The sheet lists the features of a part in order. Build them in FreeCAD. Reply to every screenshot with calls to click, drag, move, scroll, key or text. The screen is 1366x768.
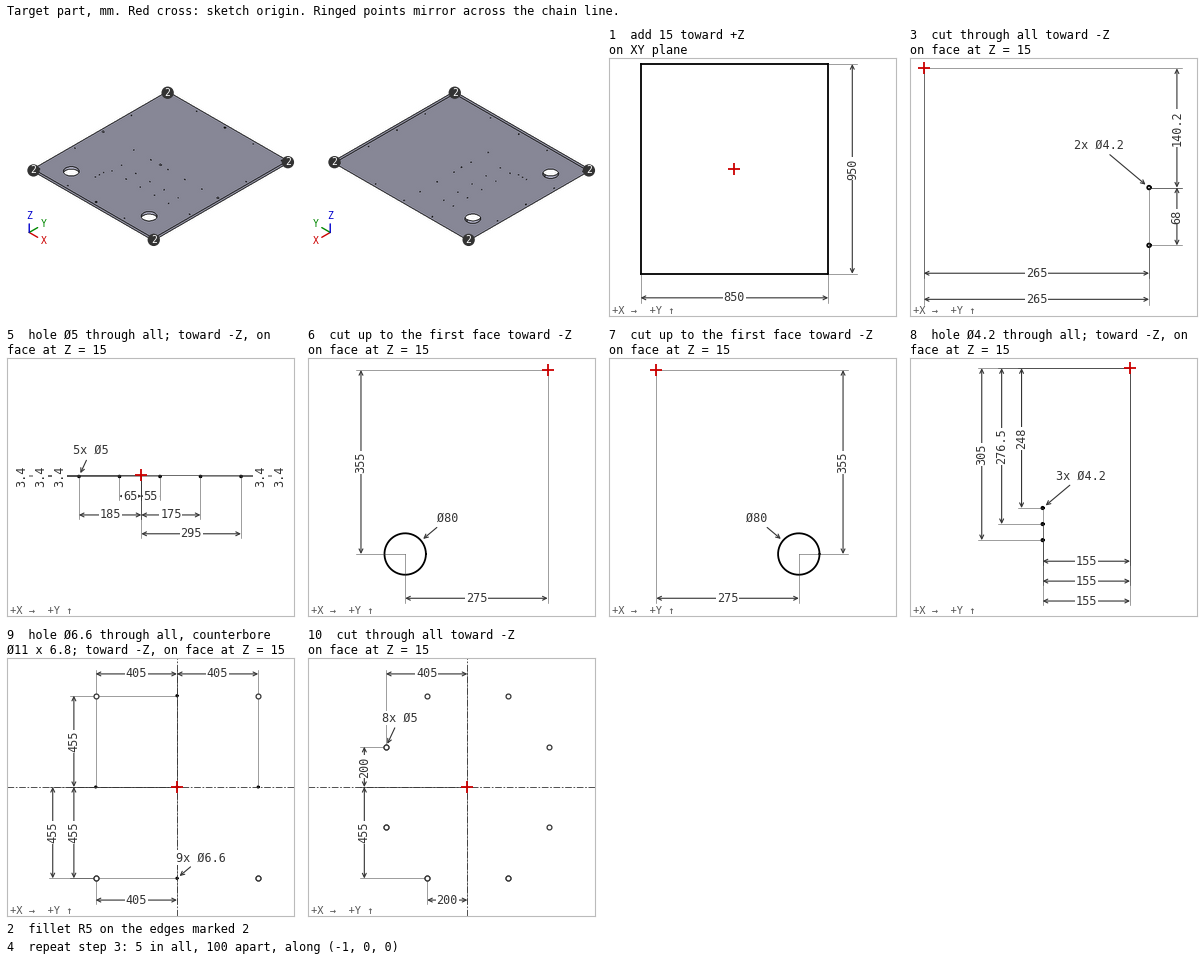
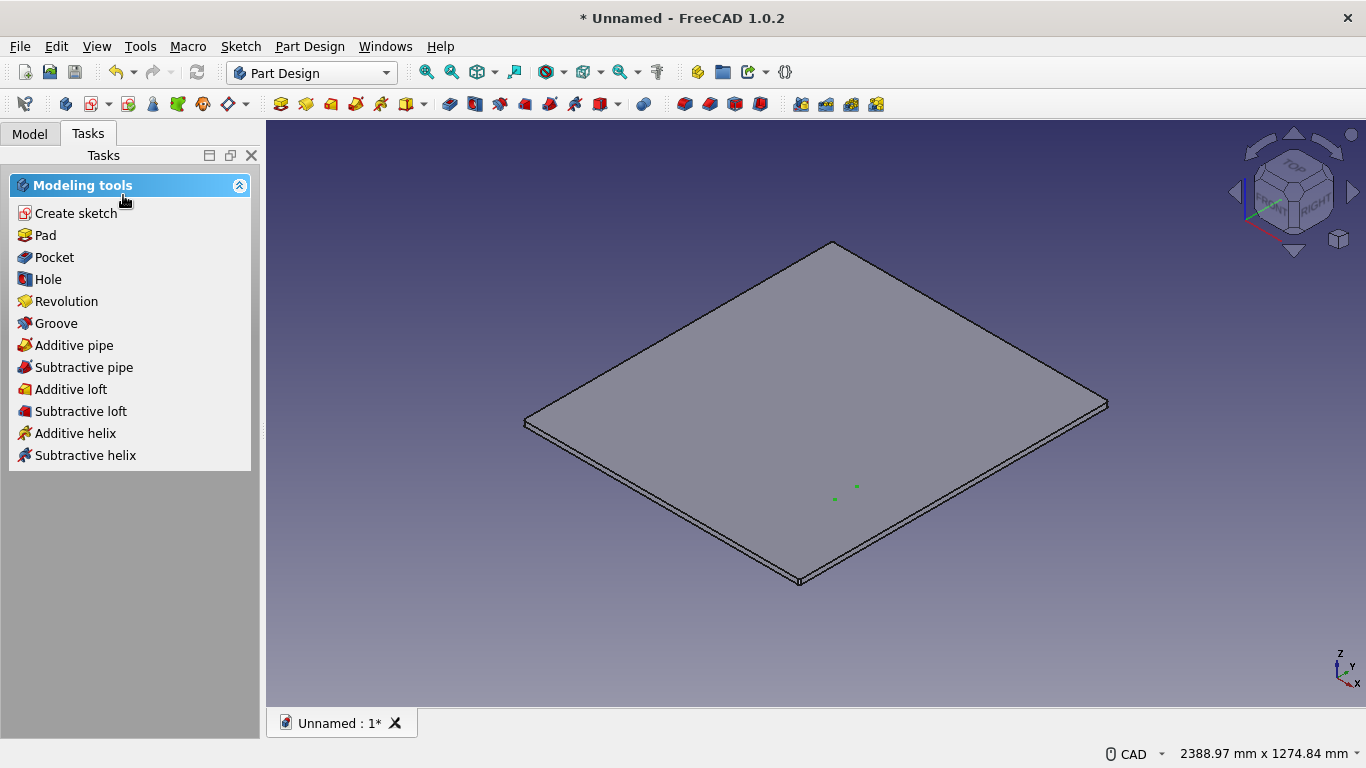
click(450, 104)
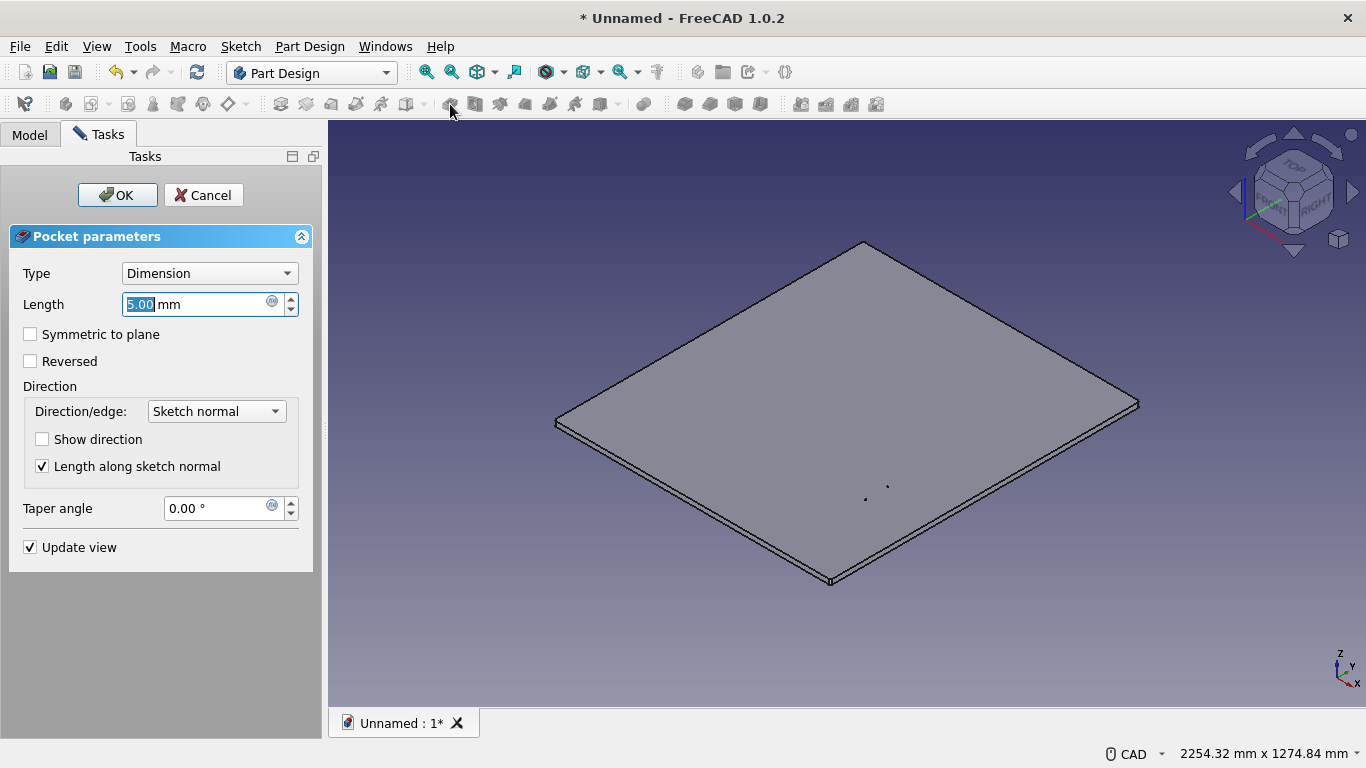
click(210, 274)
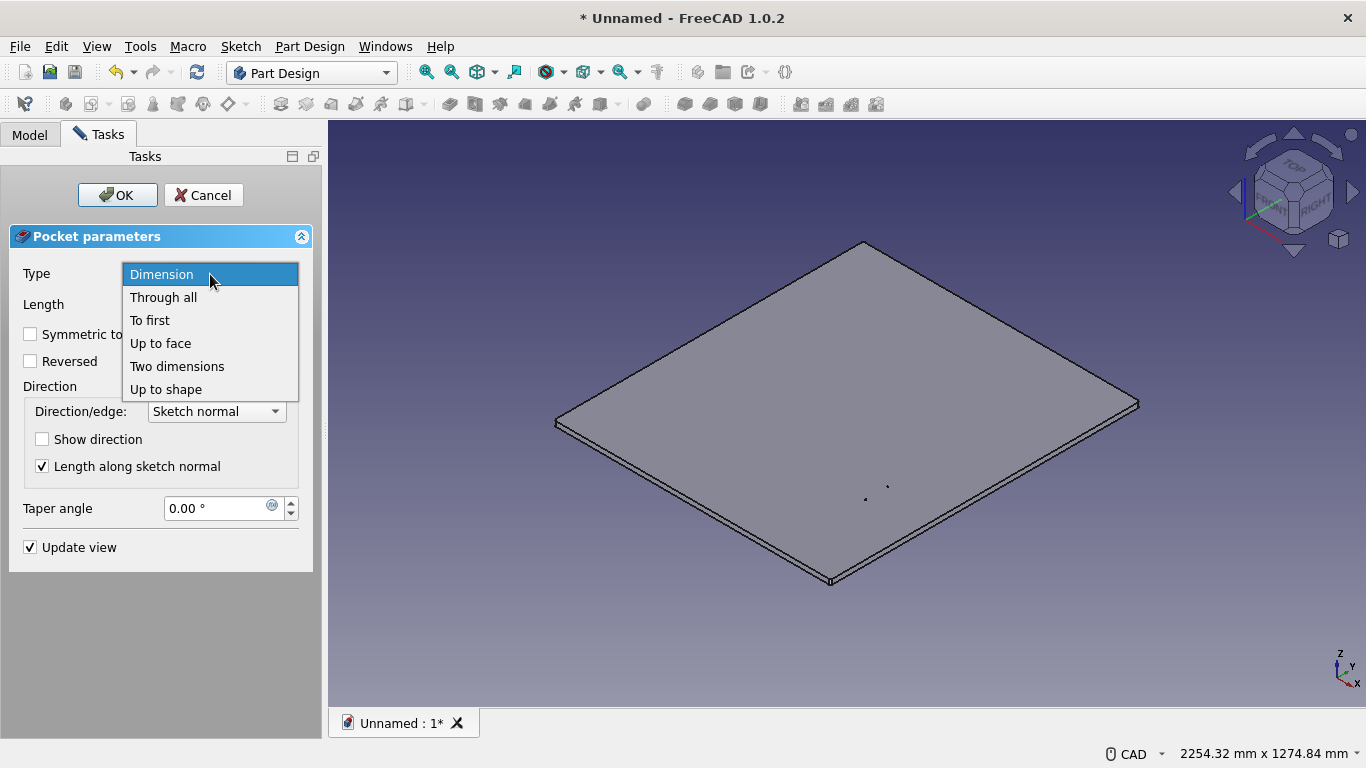
click(208, 298)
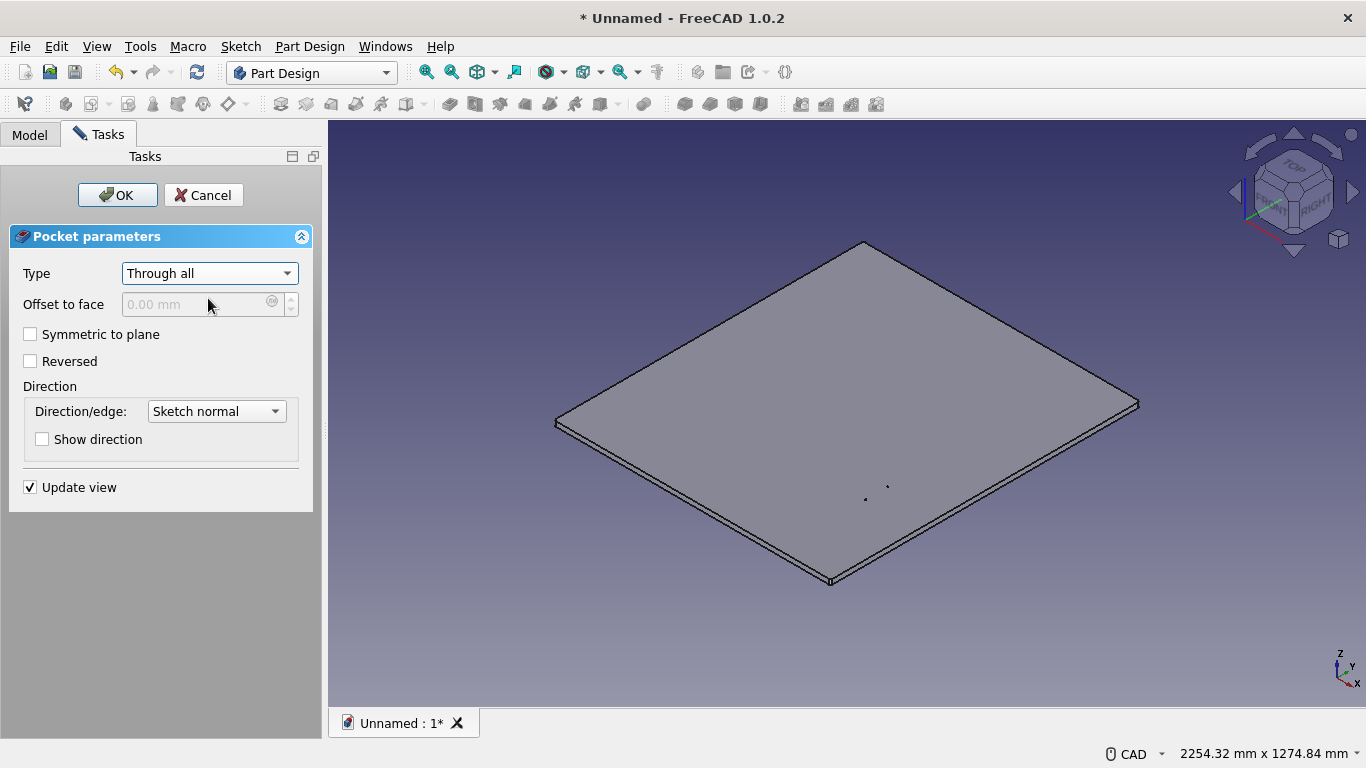
click(118, 195)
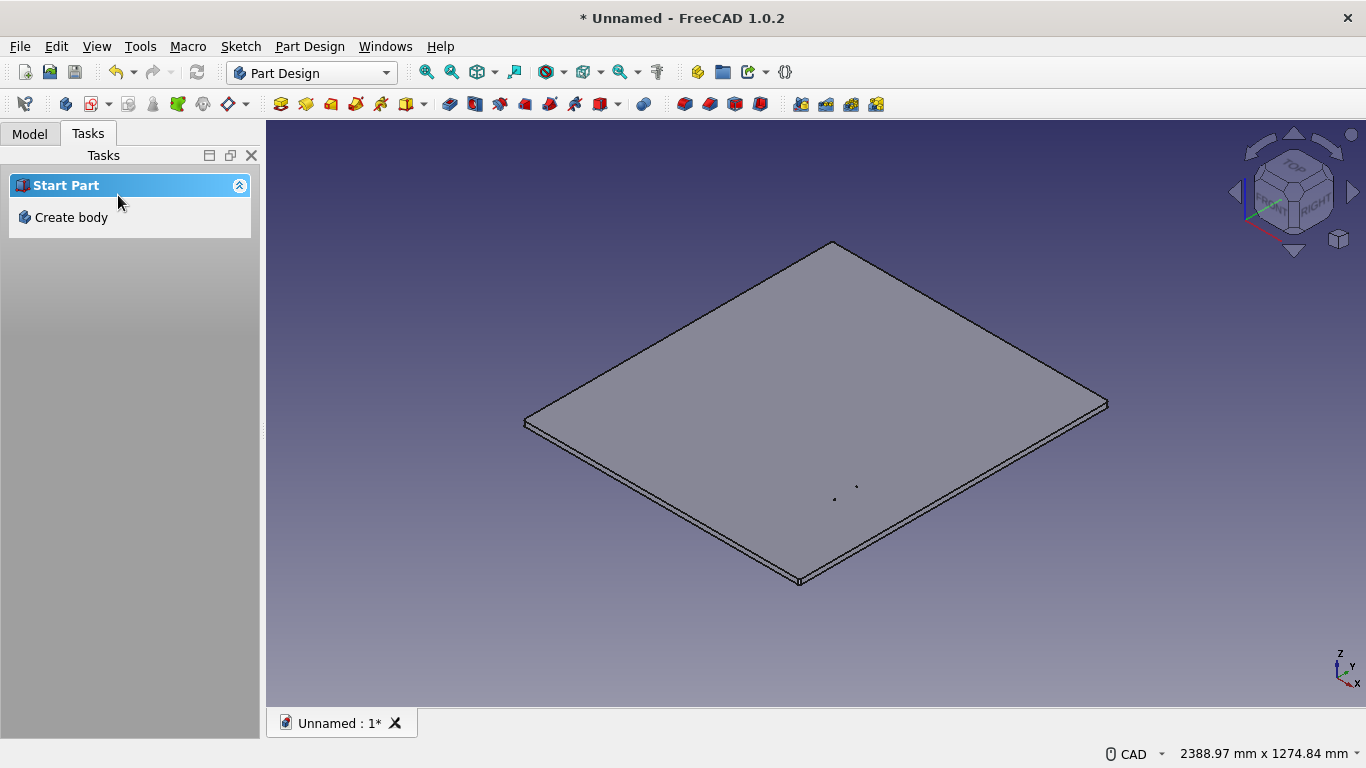
click(30, 134)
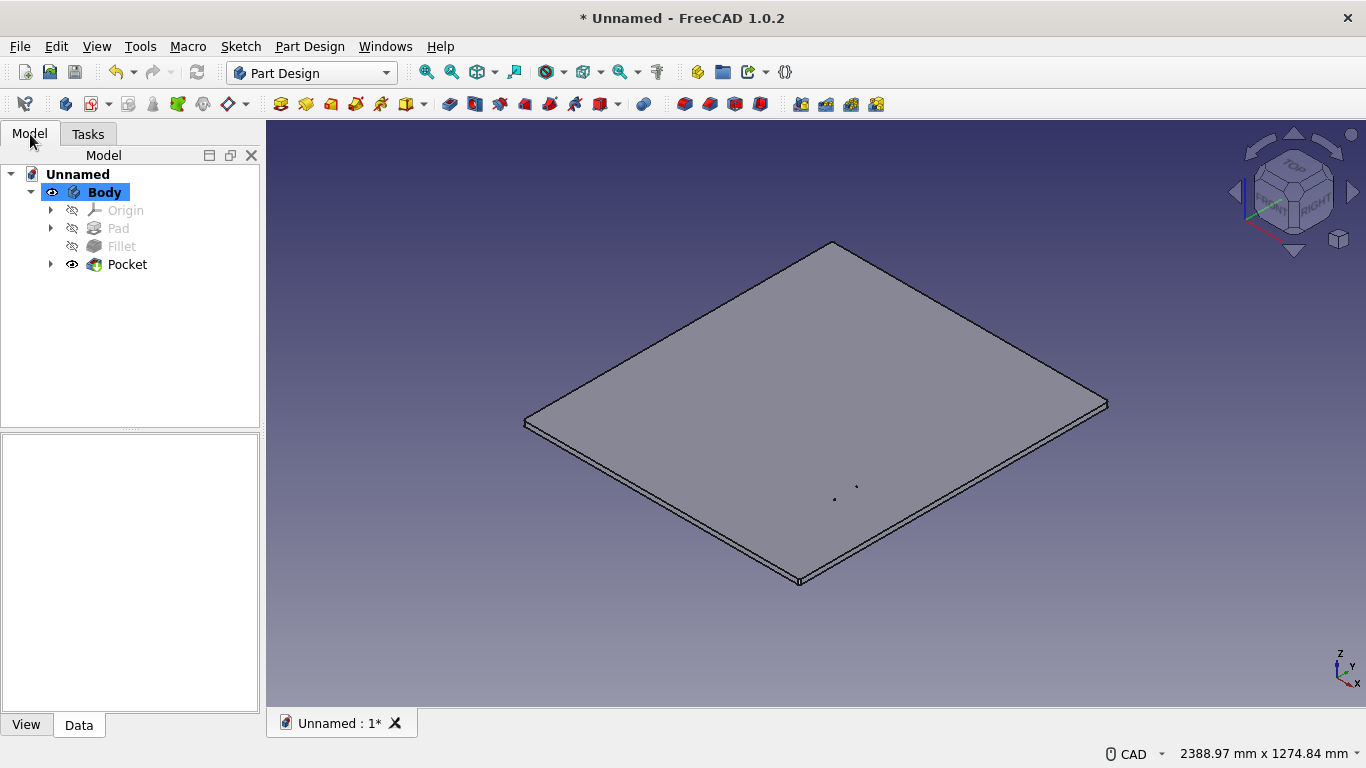
click(117, 264)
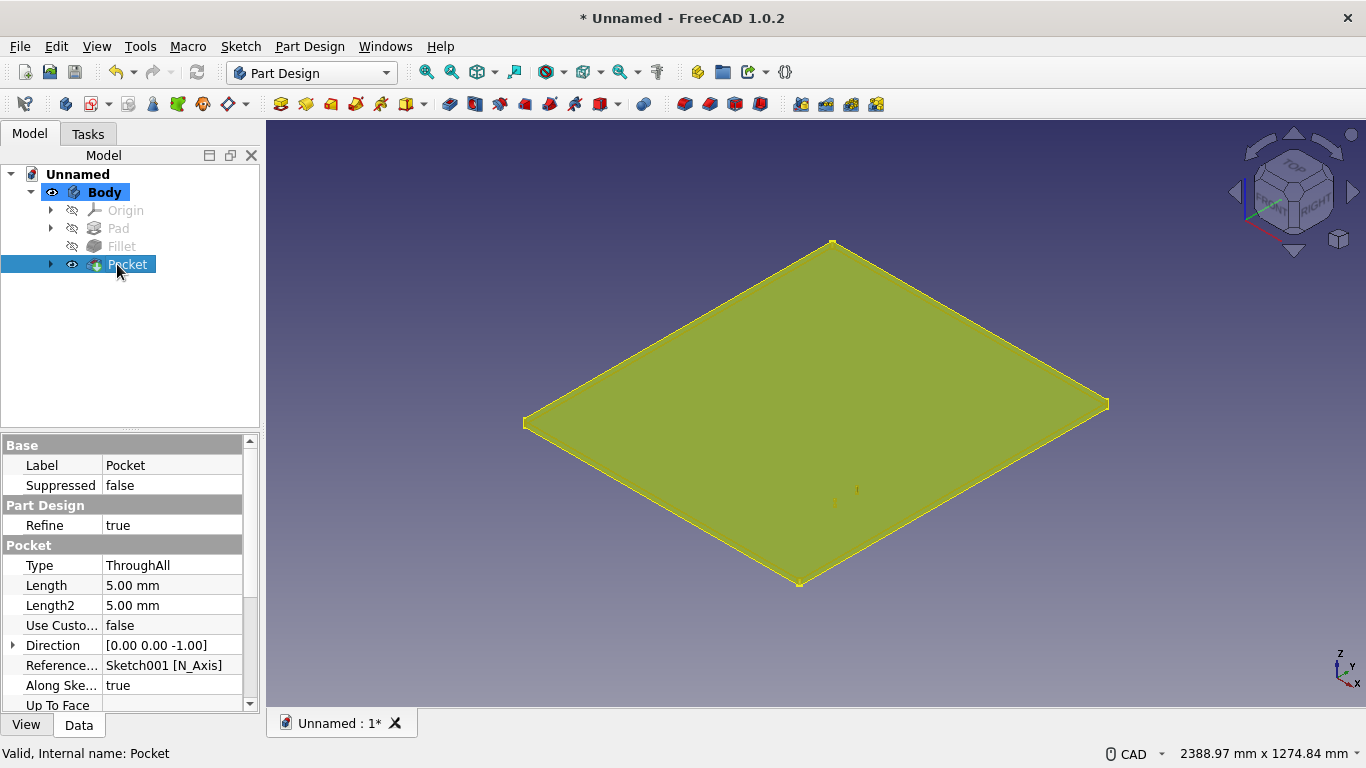
click(826, 104)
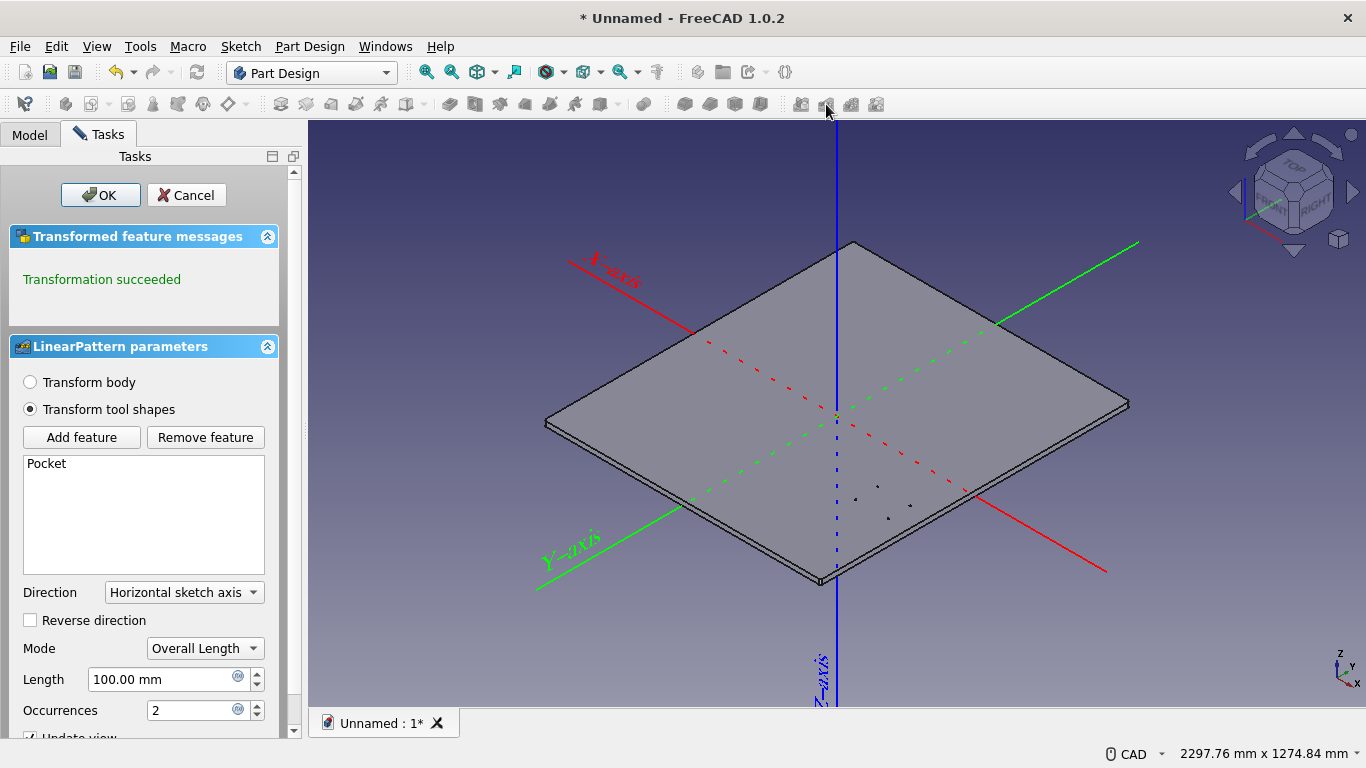
click(185, 592)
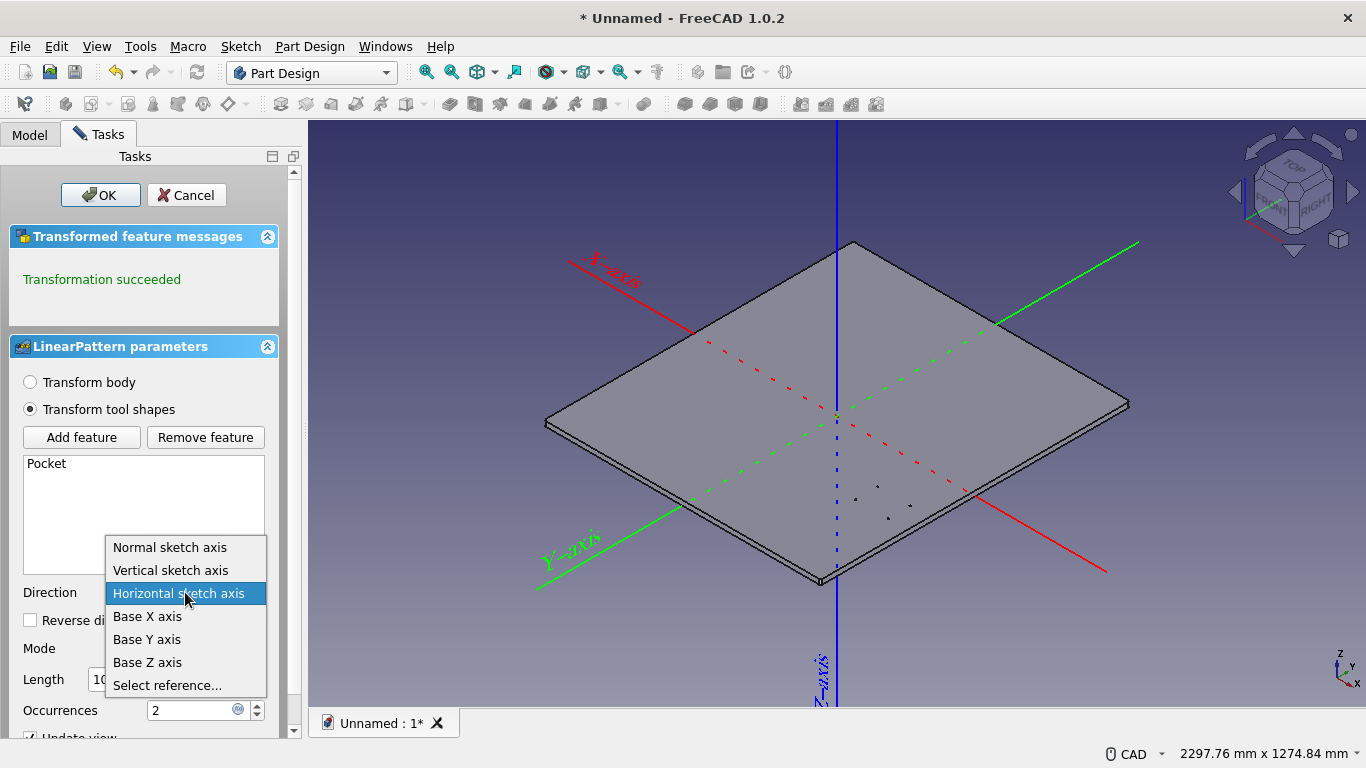
click(184, 616)